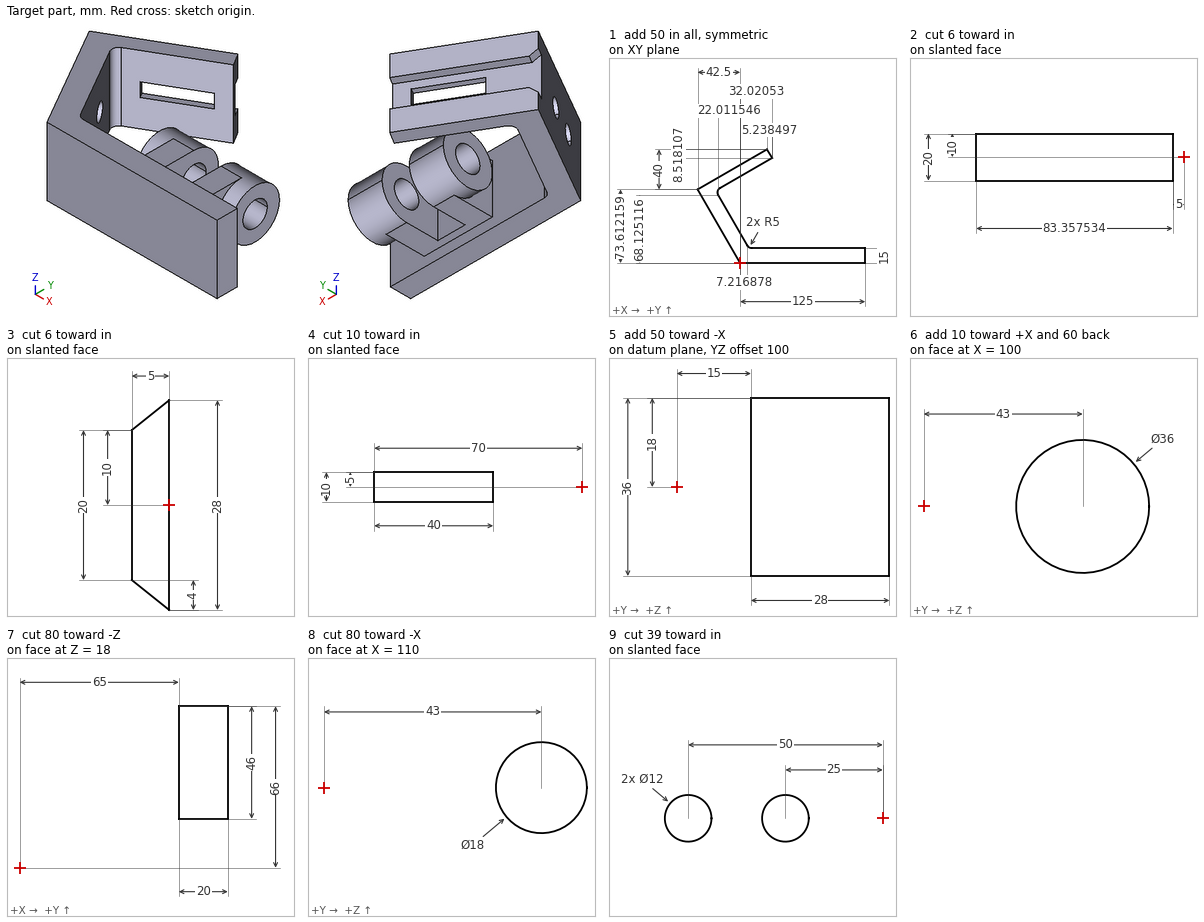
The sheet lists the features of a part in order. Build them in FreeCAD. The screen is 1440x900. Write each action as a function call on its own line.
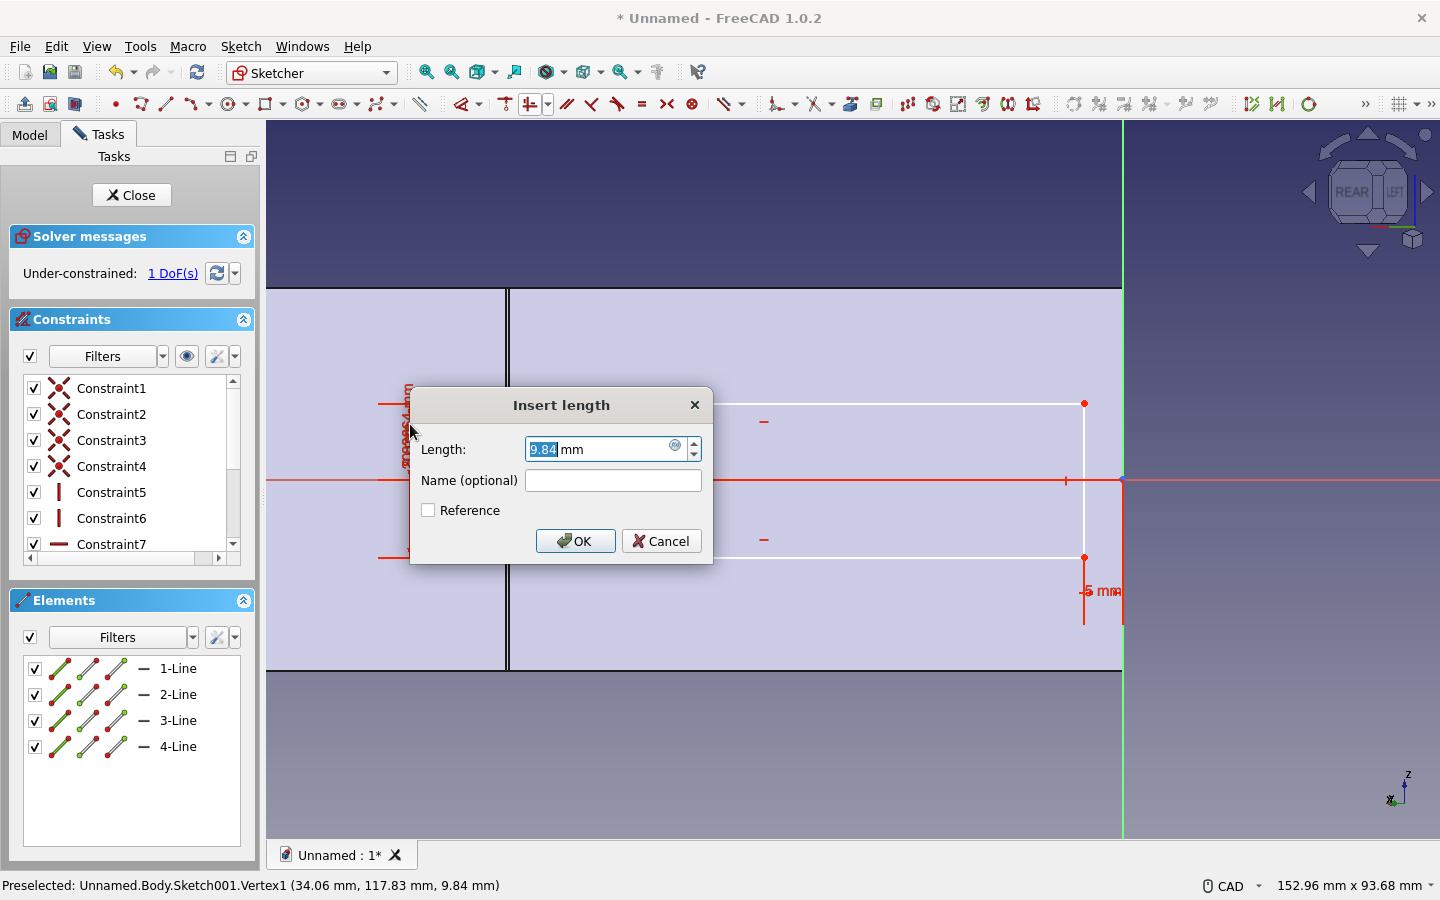
text(10)
key(Return)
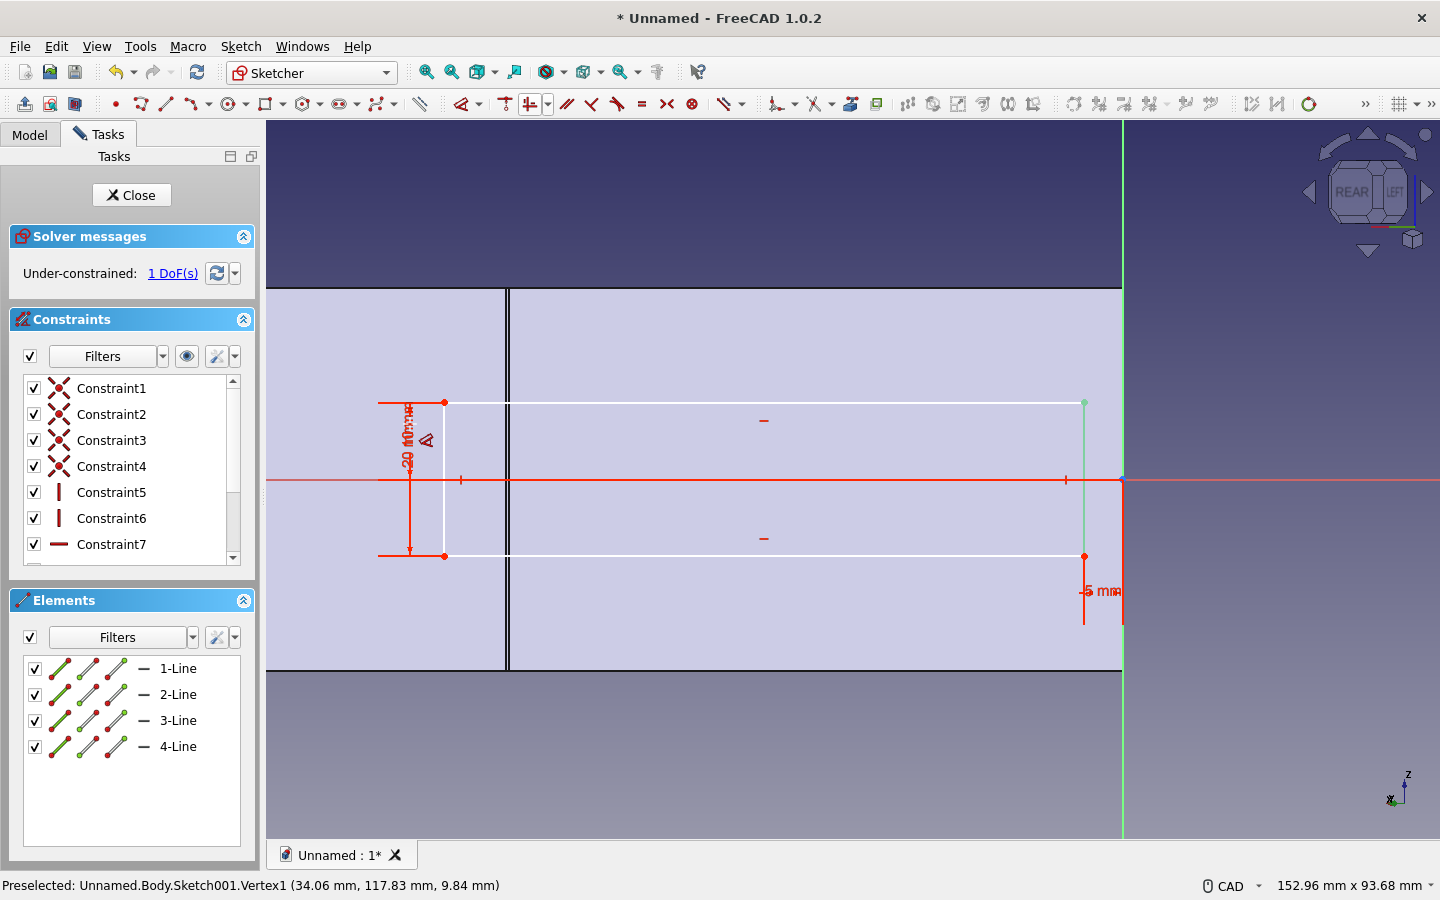
click(636, 556)
click(764, 590)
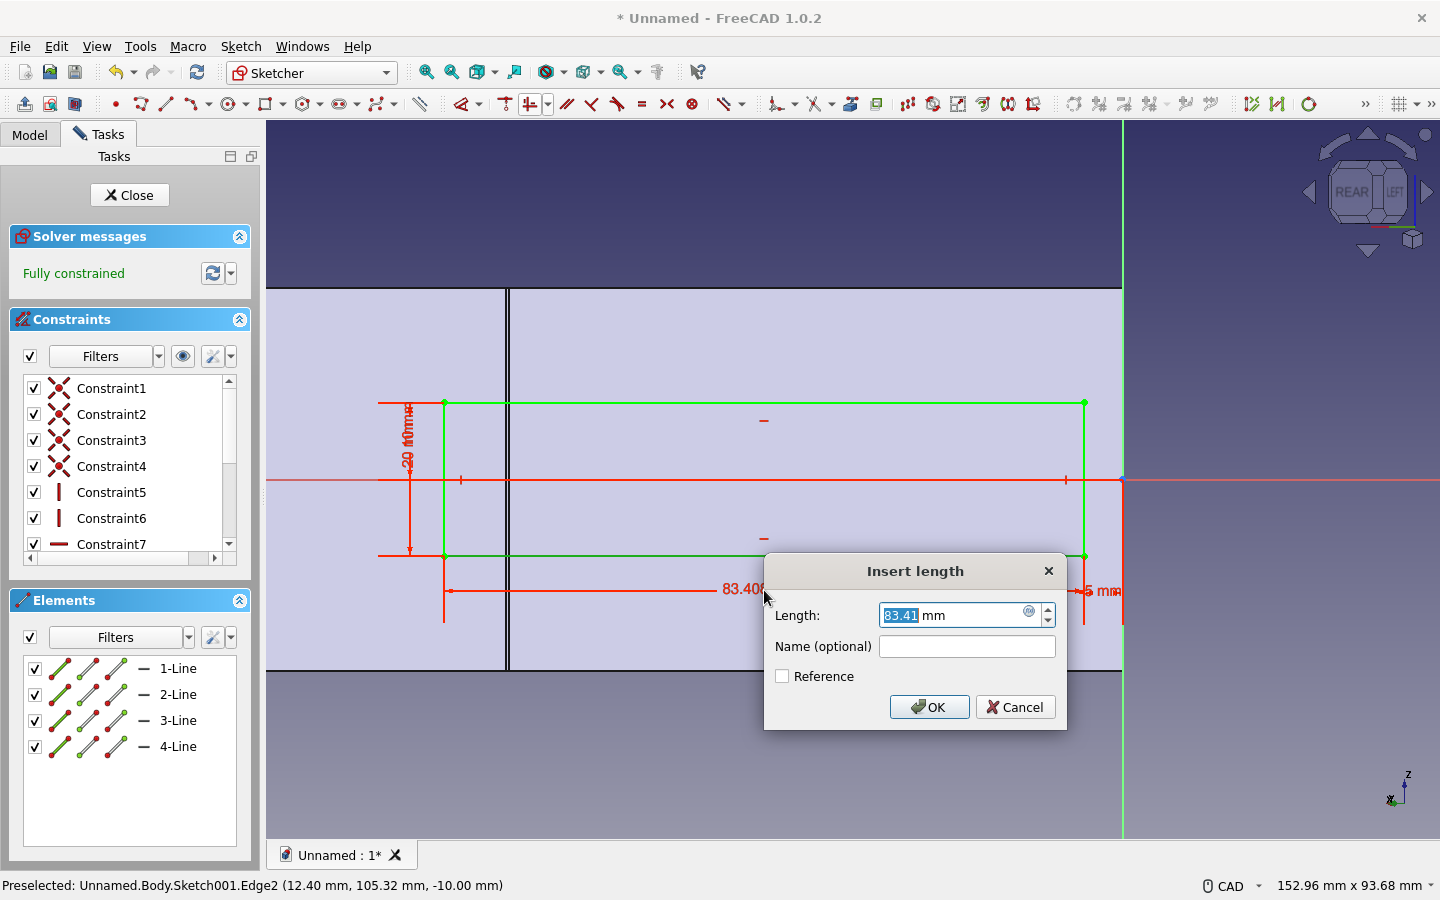
text(83.357534)
key(Return)
key(Escape)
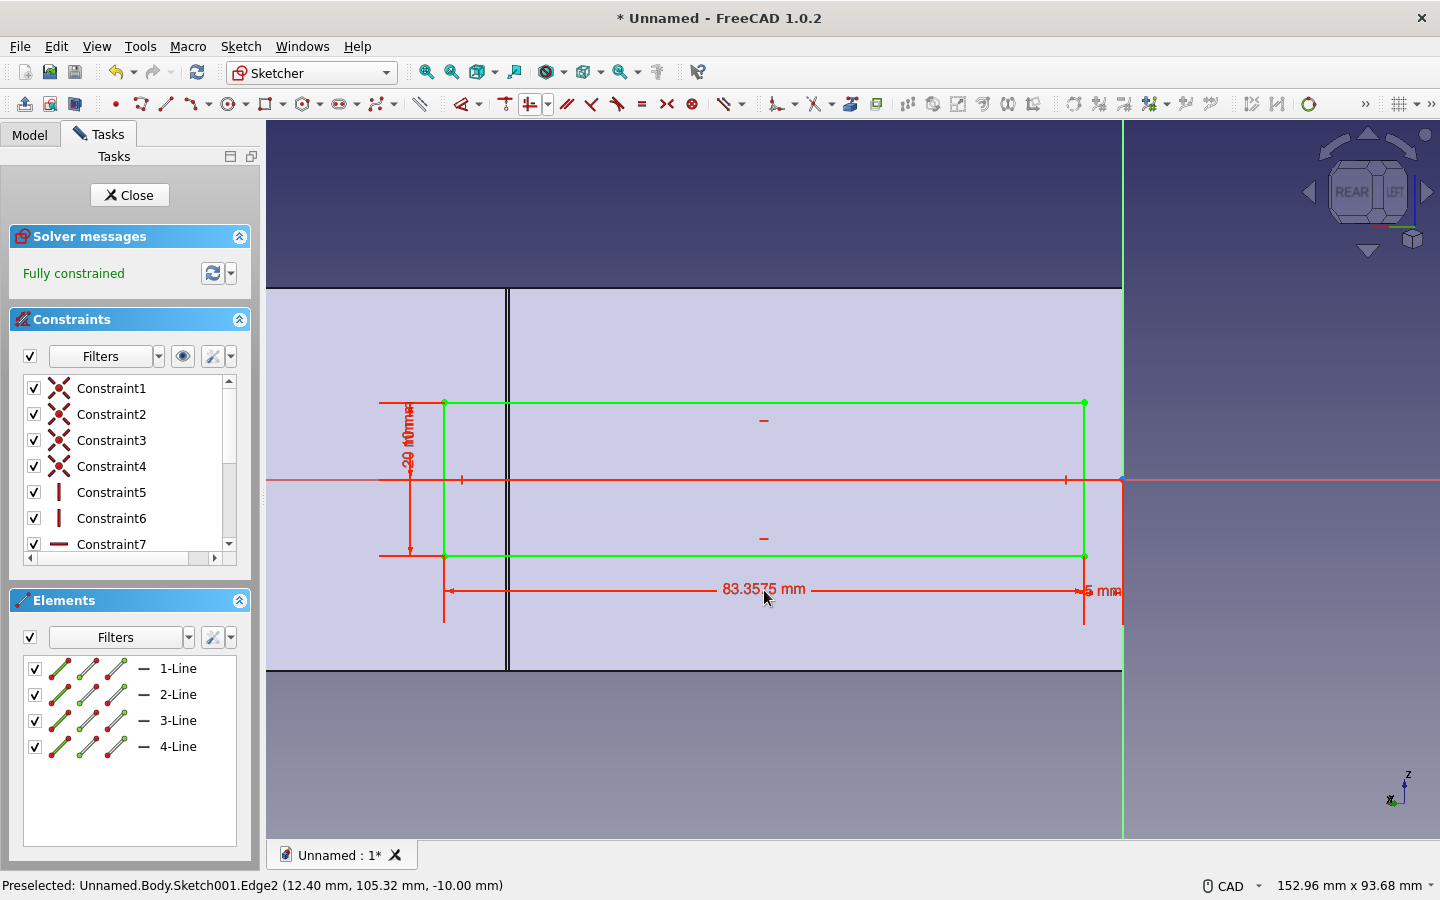
click(130, 195)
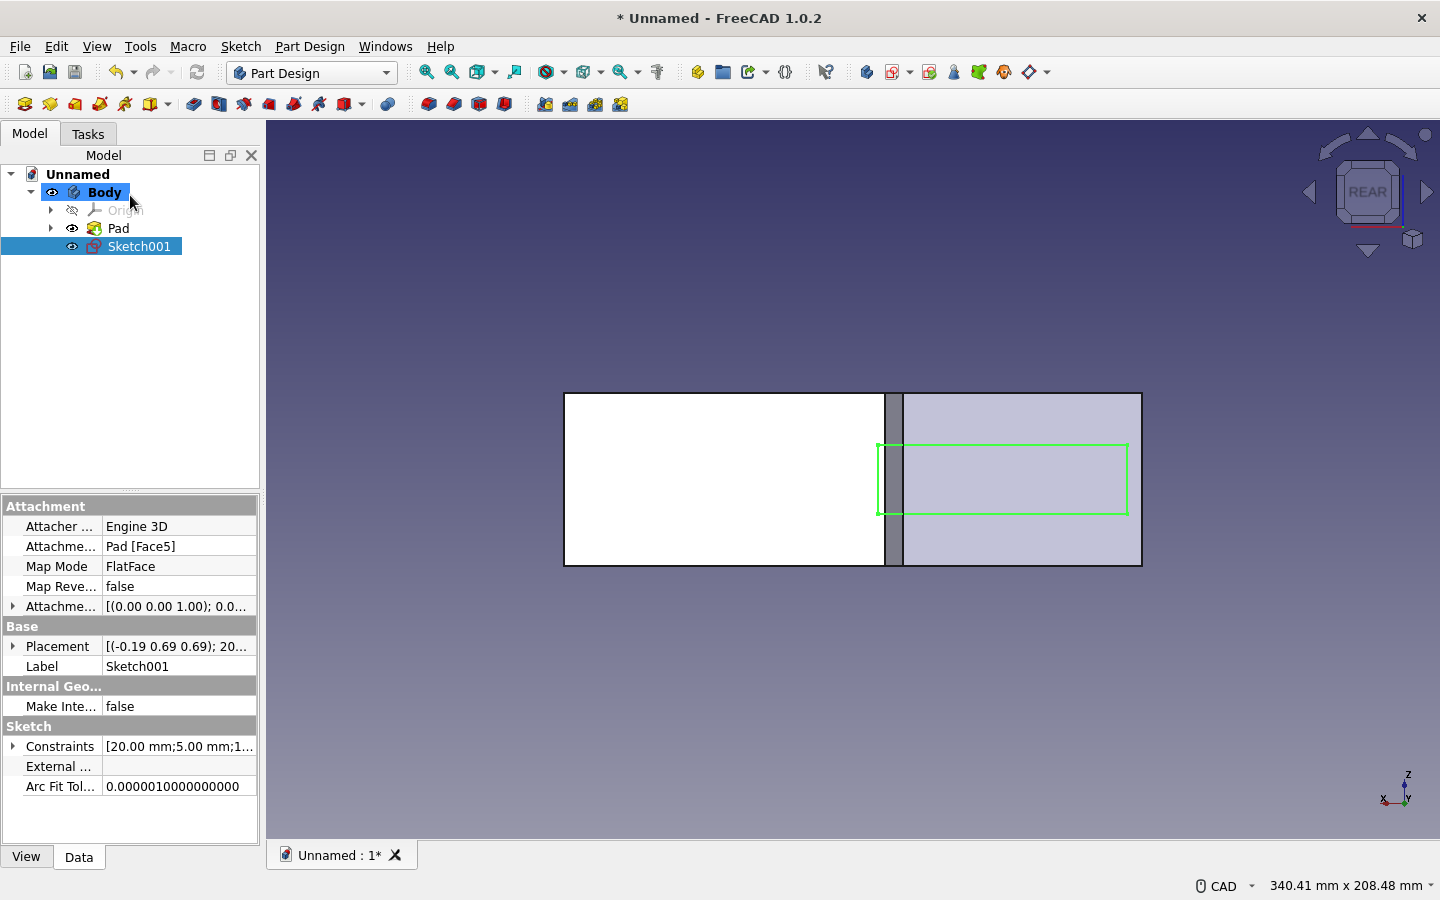
click(194, 104)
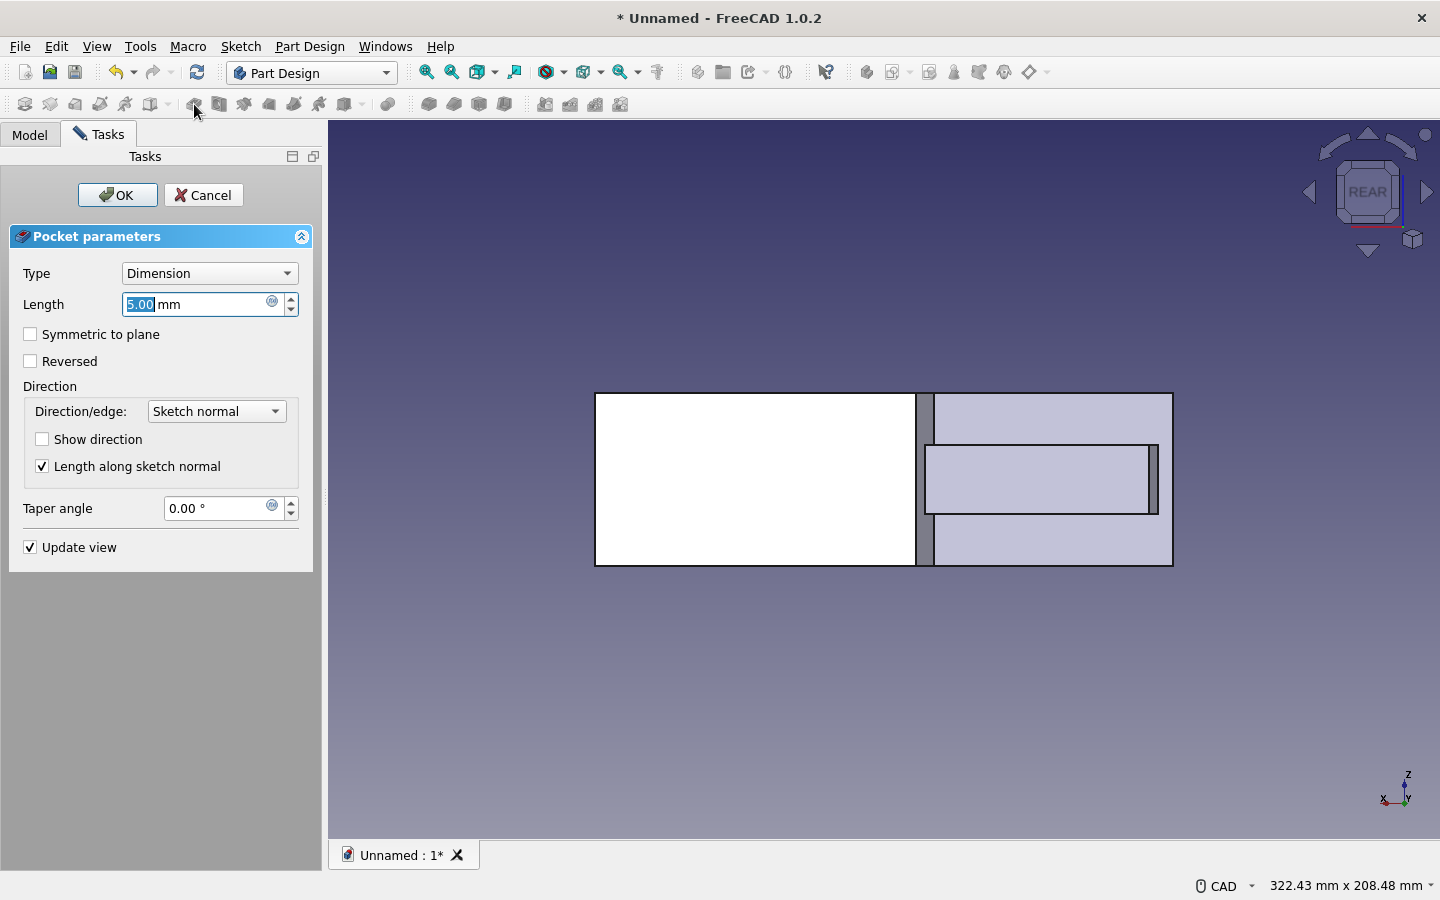
text(6)
key(Tab)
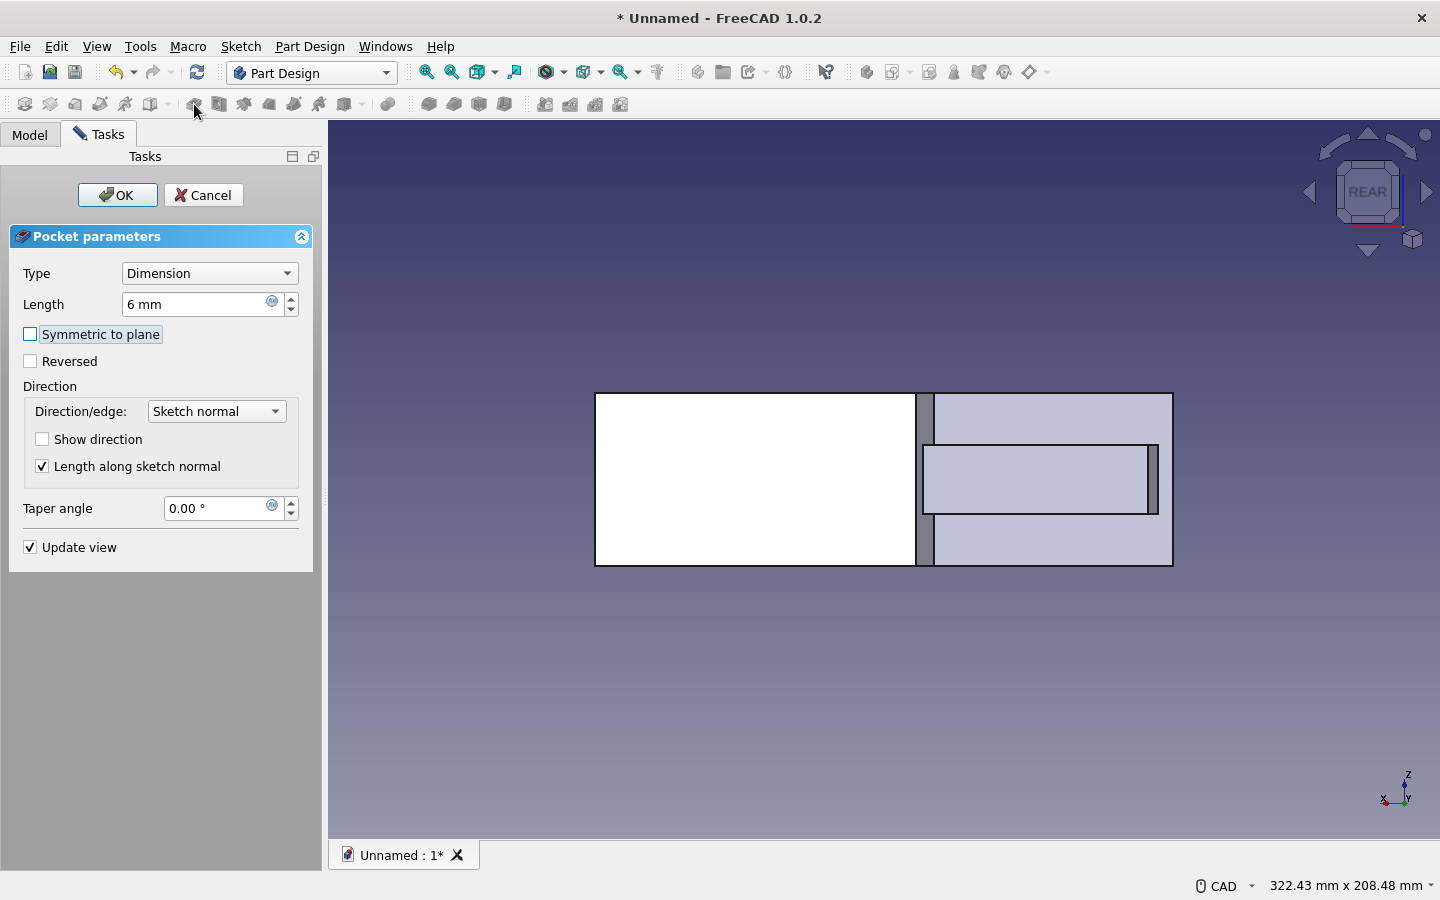
click(118, 195)